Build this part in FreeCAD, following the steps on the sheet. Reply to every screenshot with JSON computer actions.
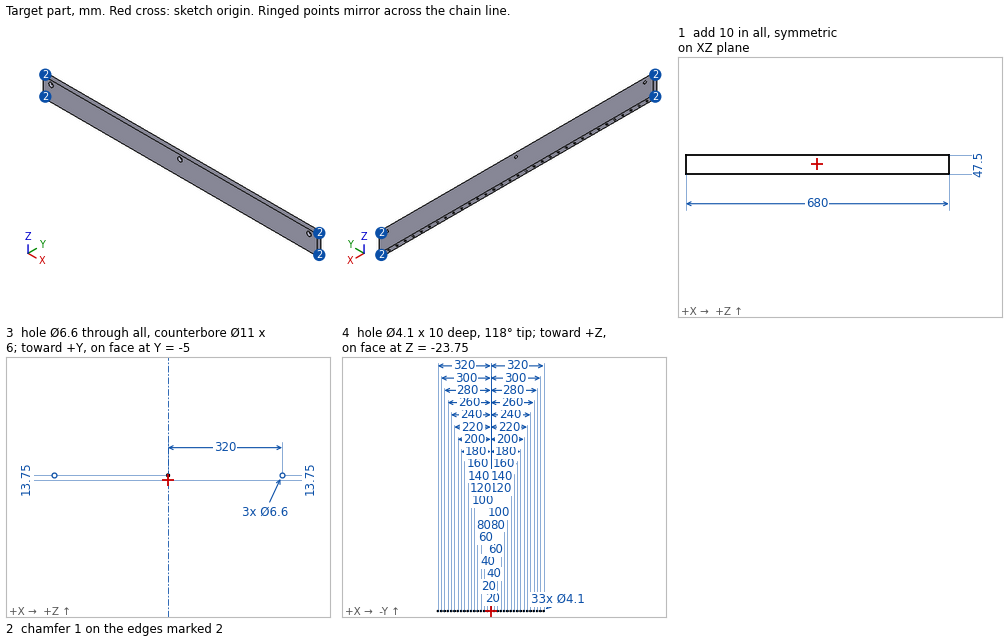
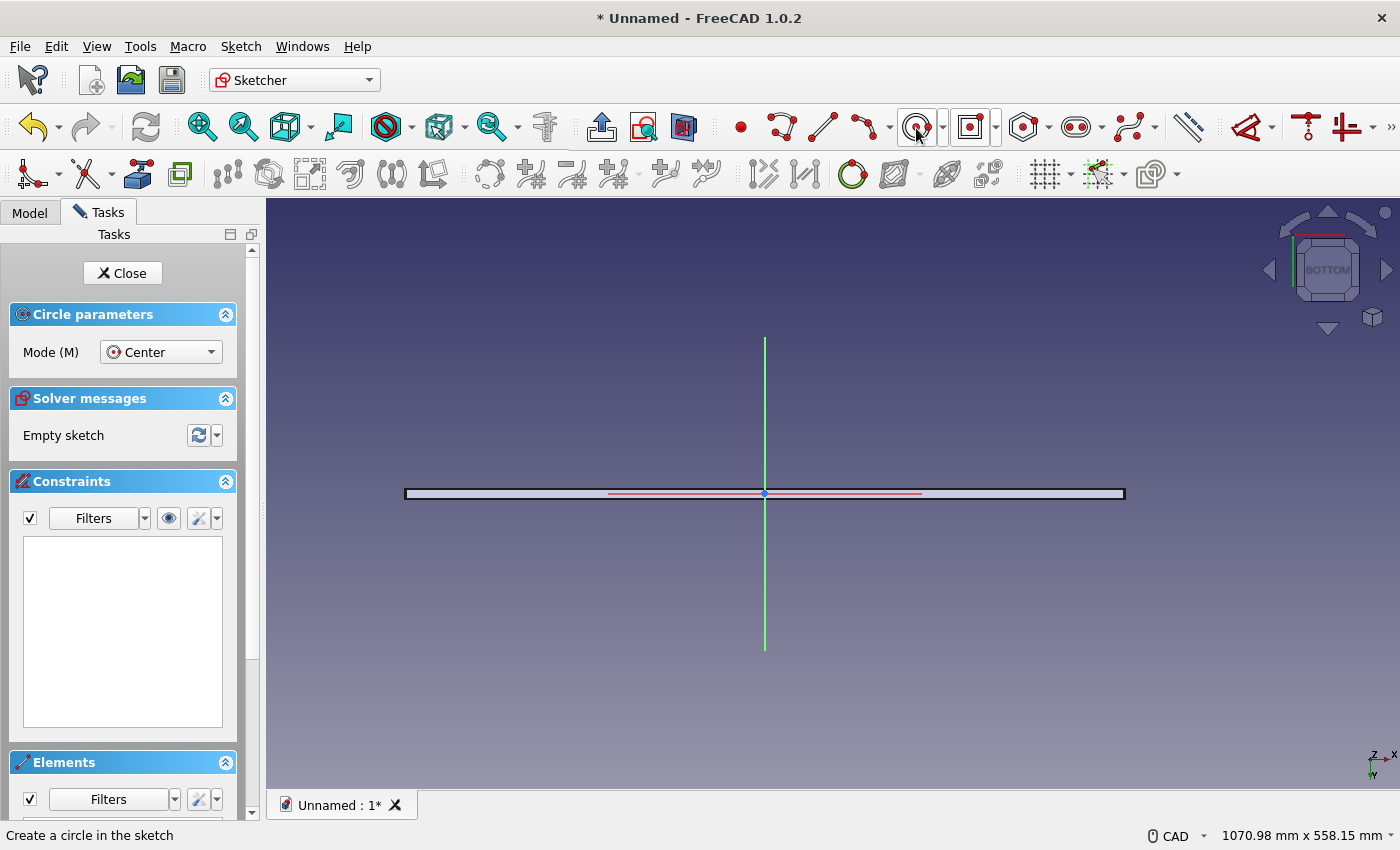
{"action": "scroll", "coordinate": [1104, 494], "scroll_direction": "up", "scroll_amount": 12}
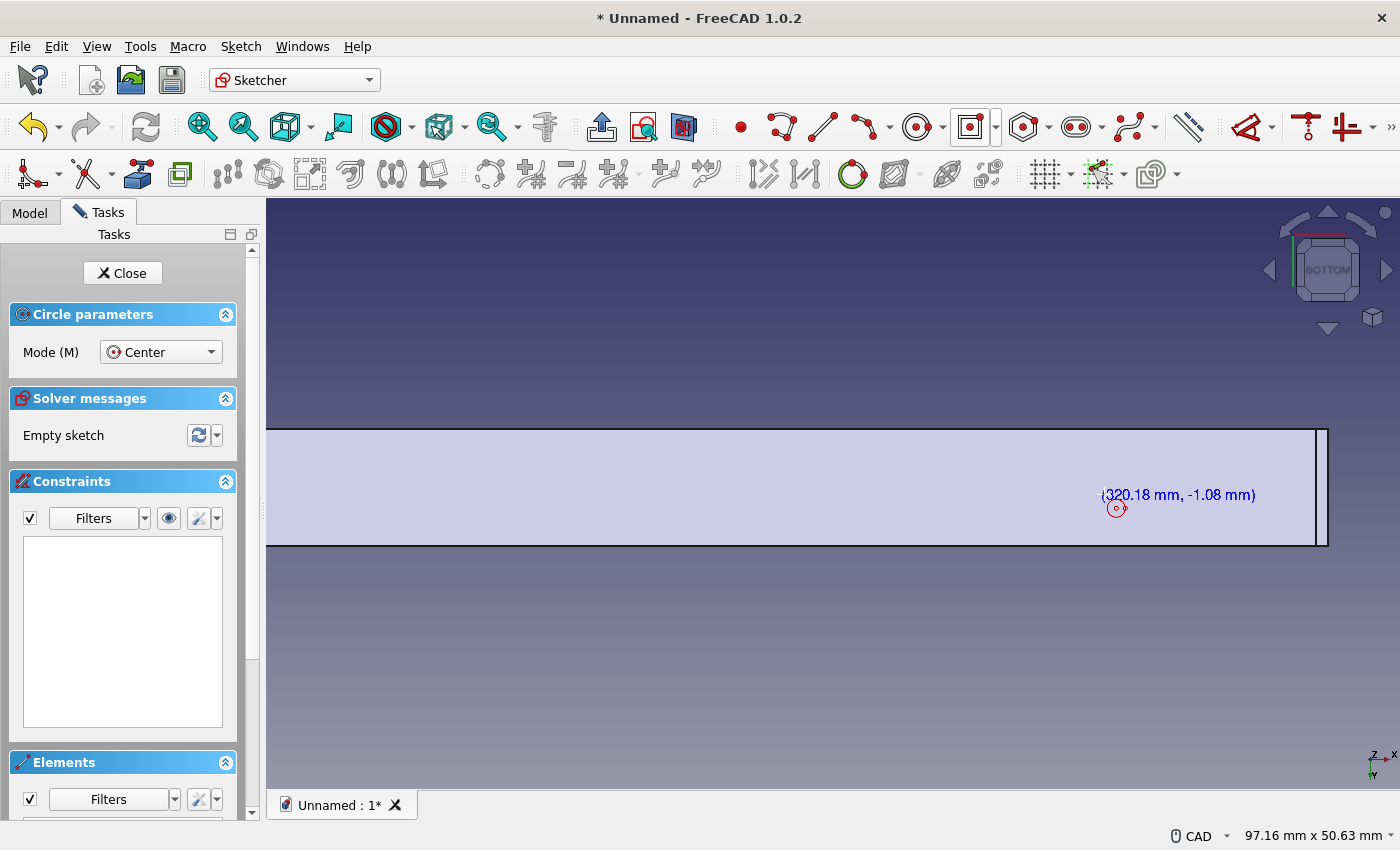
{"action": "scroll", "coordinate": [1104, 494], "scroll_direction": "down", "scroll_amount": 12}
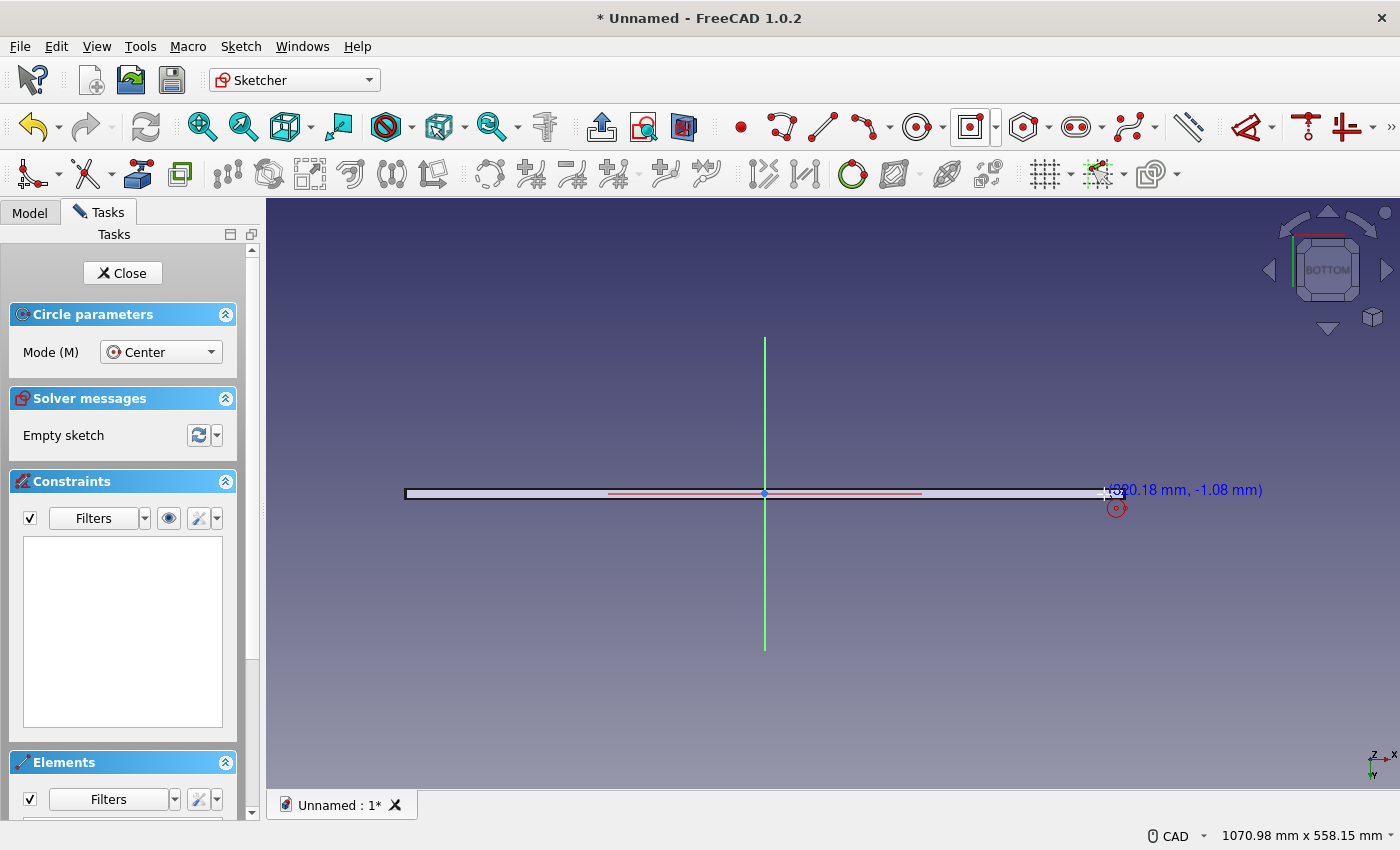
{"action": "left_click", "coordinate": [1104, 494]}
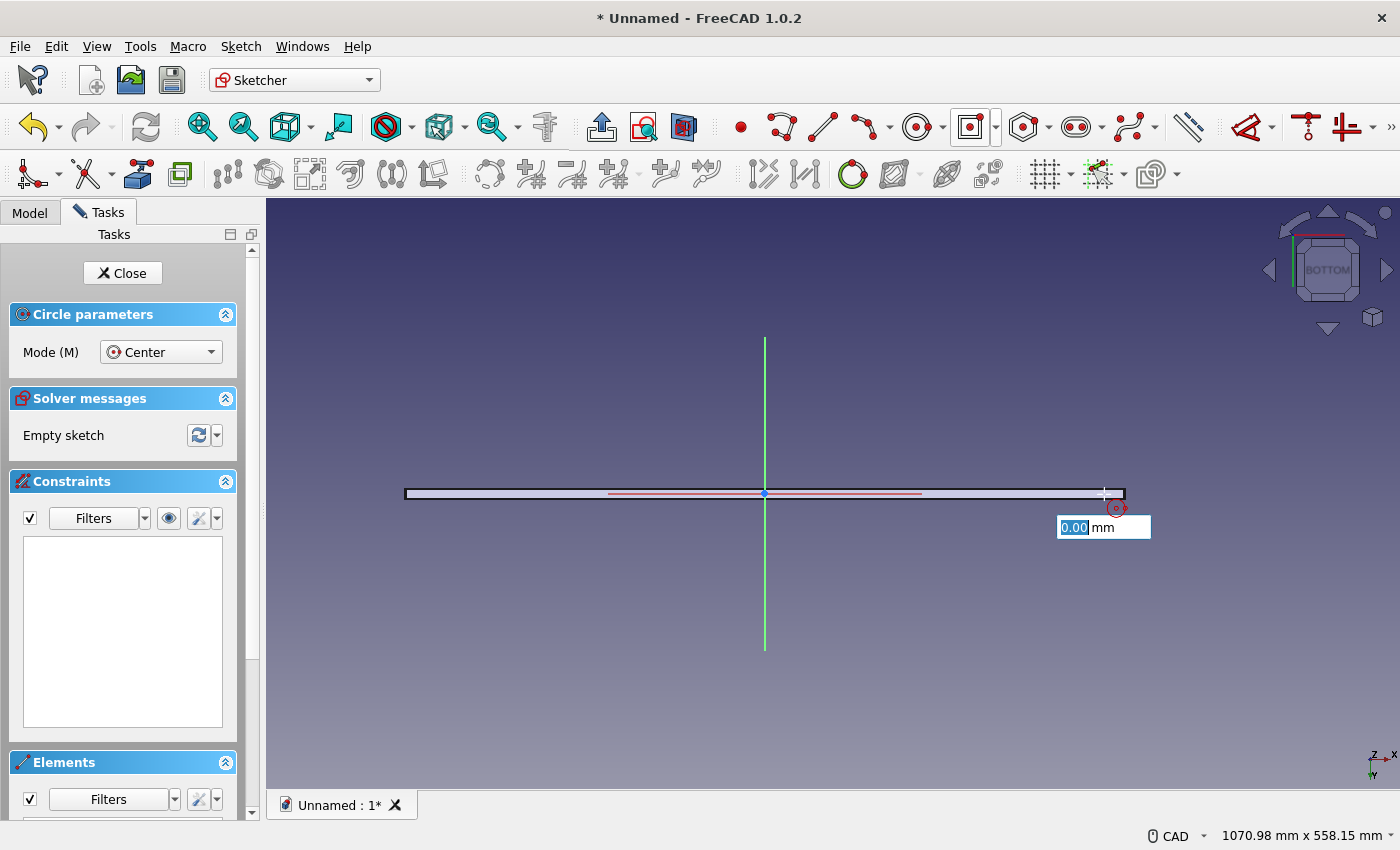
{"action": "scroll", "coordinate": [1103, 496], "scroll_direction": "up", "scroll_amount": 11}
{"action": "mouse_move", "coordinate": [1098, 491]}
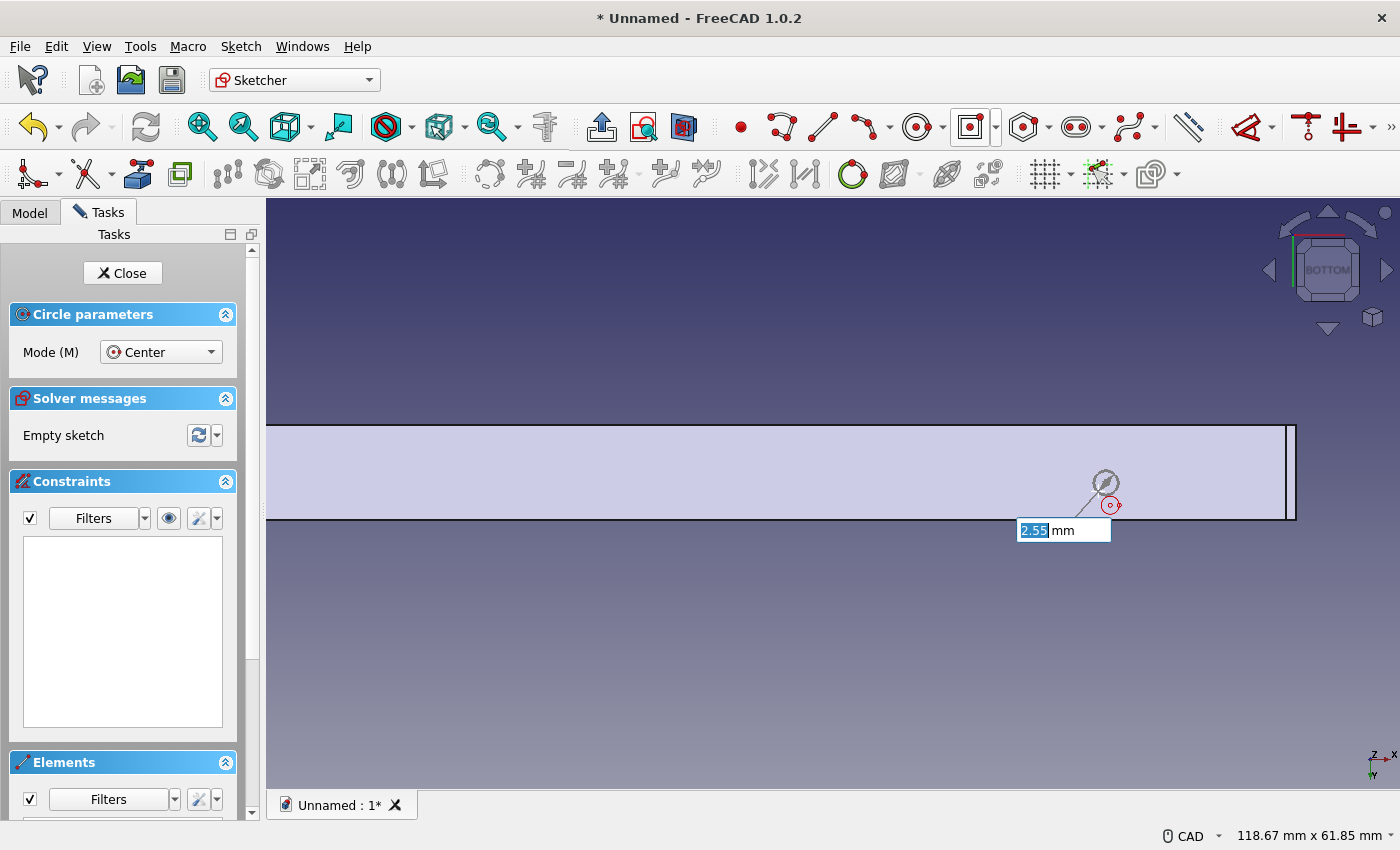
{"action": "type", "text": "4.1"}
{"action": "key", "text": "Return"}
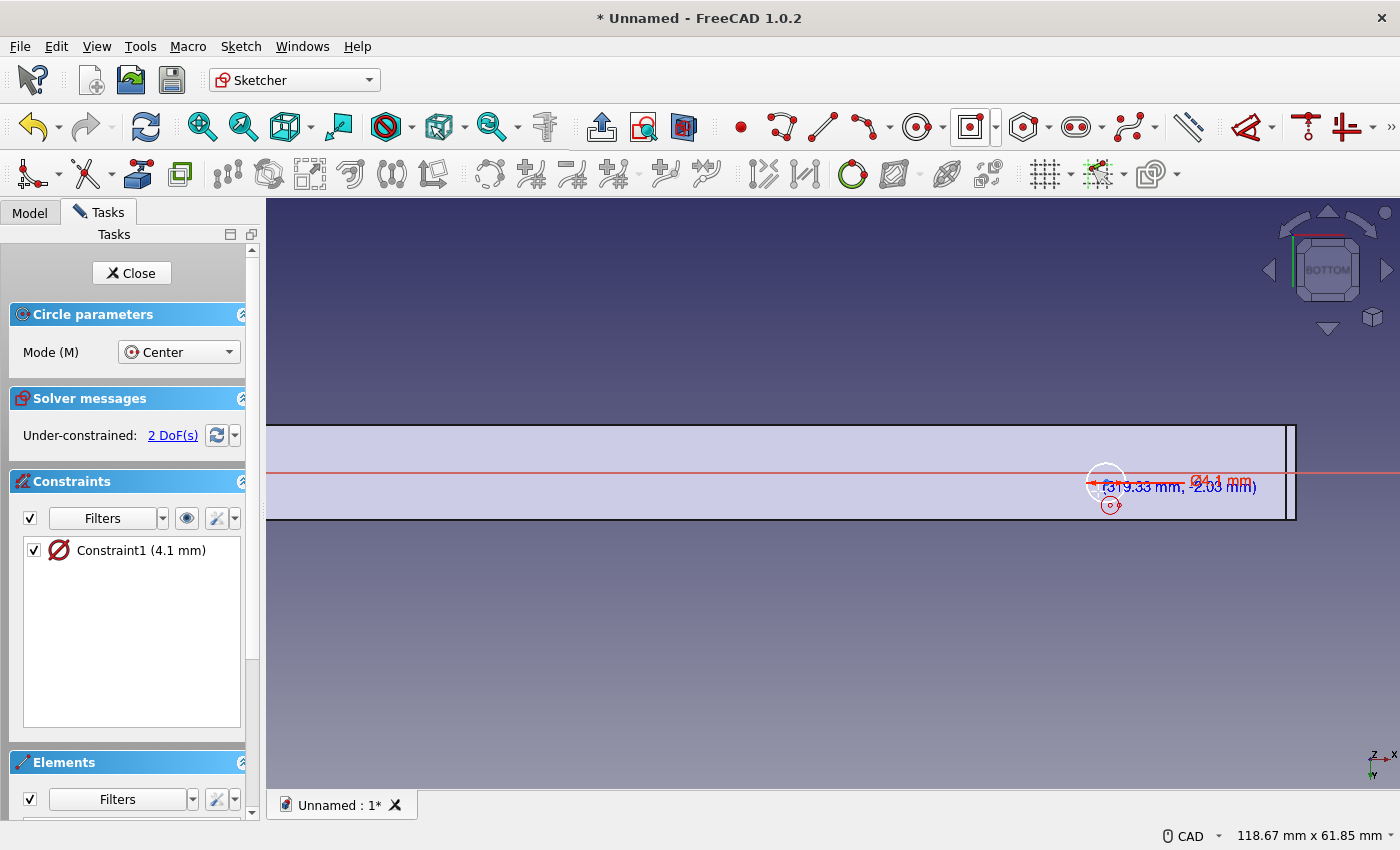
{"action": "scroll", "coordinate": [1103, 496], "scroll_direction": "down", "scroll_amount": 11}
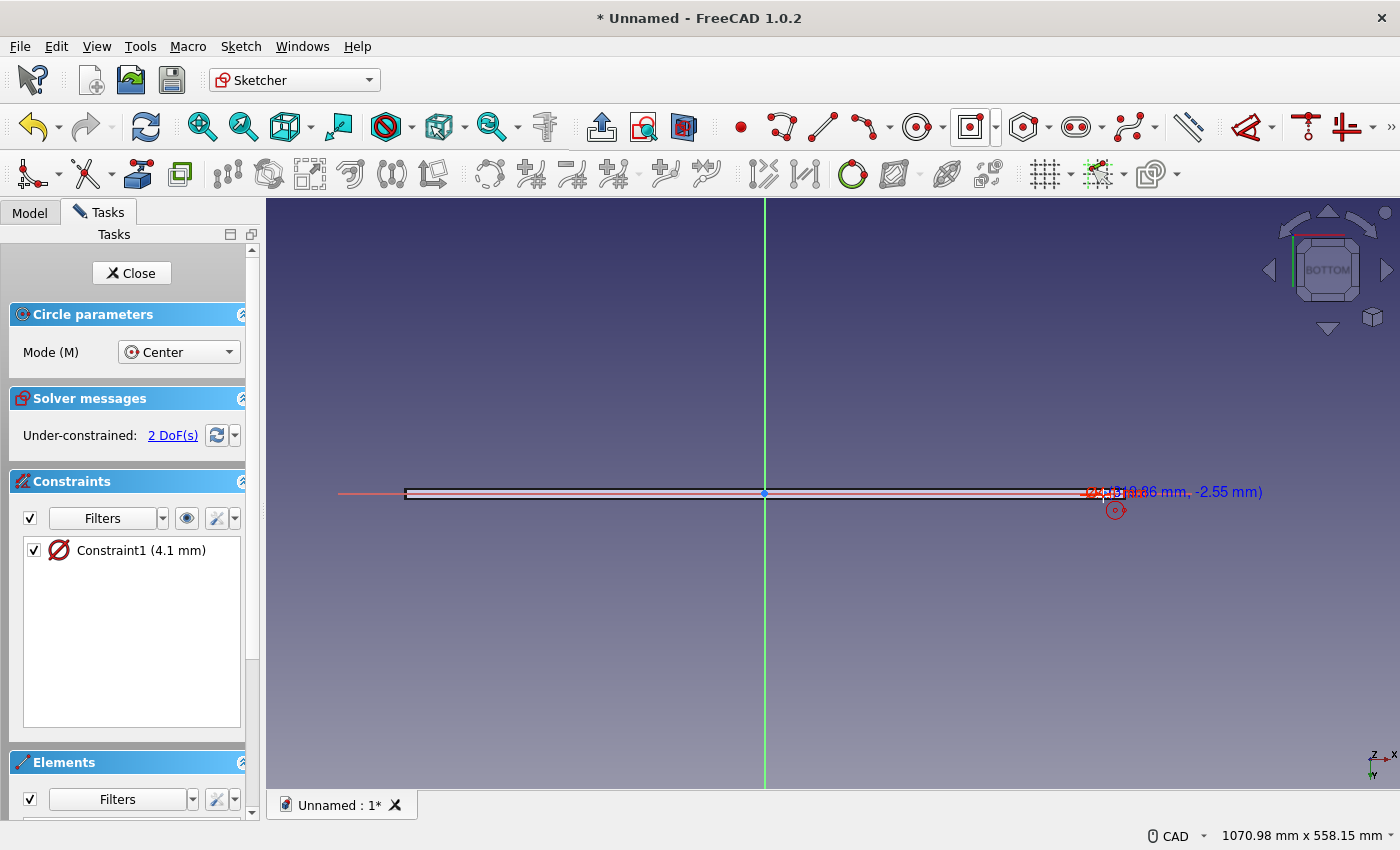
{"action": "left_click", "coordinate": [1083, 494]}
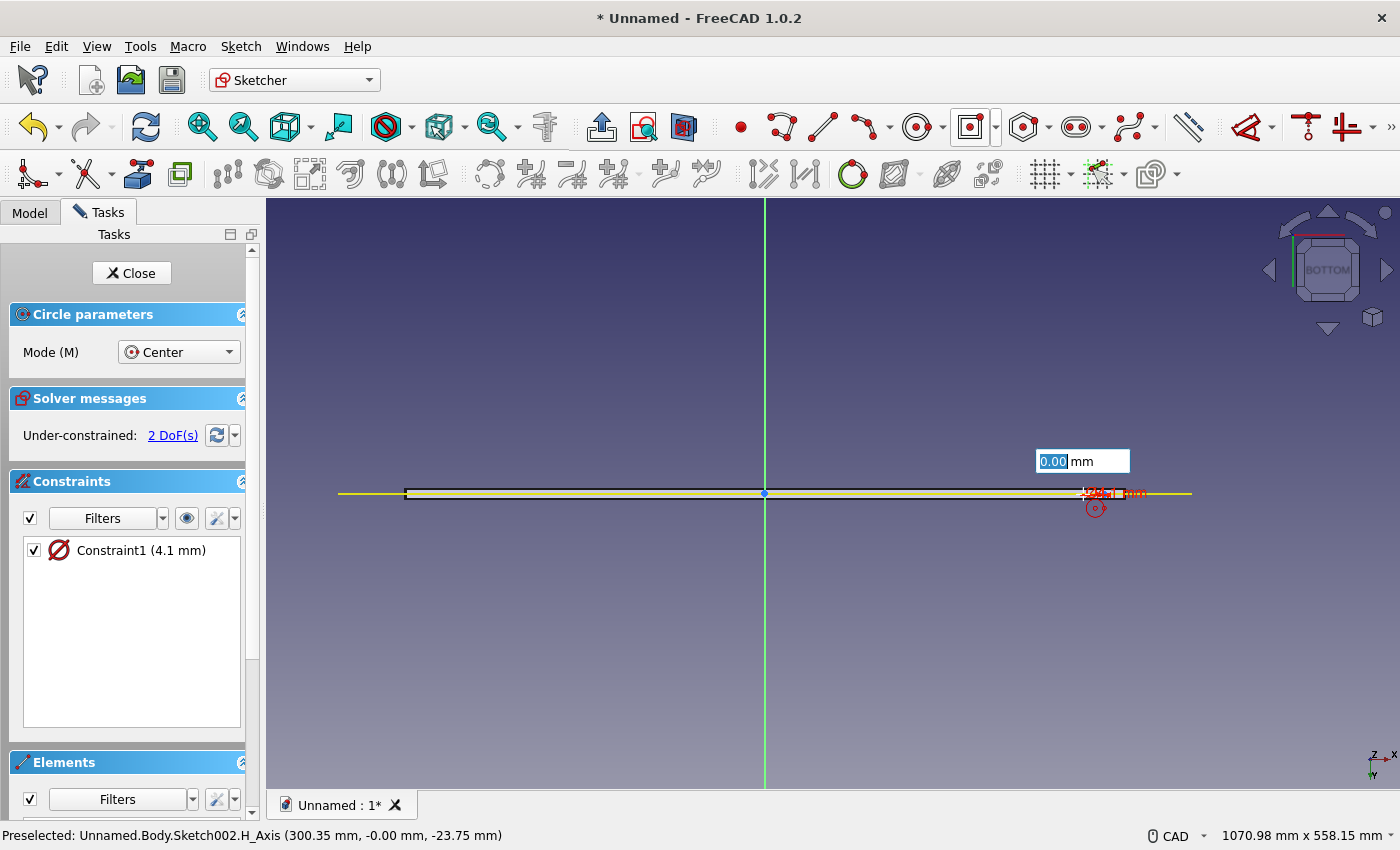
{"action": "scroll", "coordinate": [1083, 492], "scroll_direction": "up", "scroll_amount": 11}
{"action": "mouse_move", "coordinate": [1081, 486]}